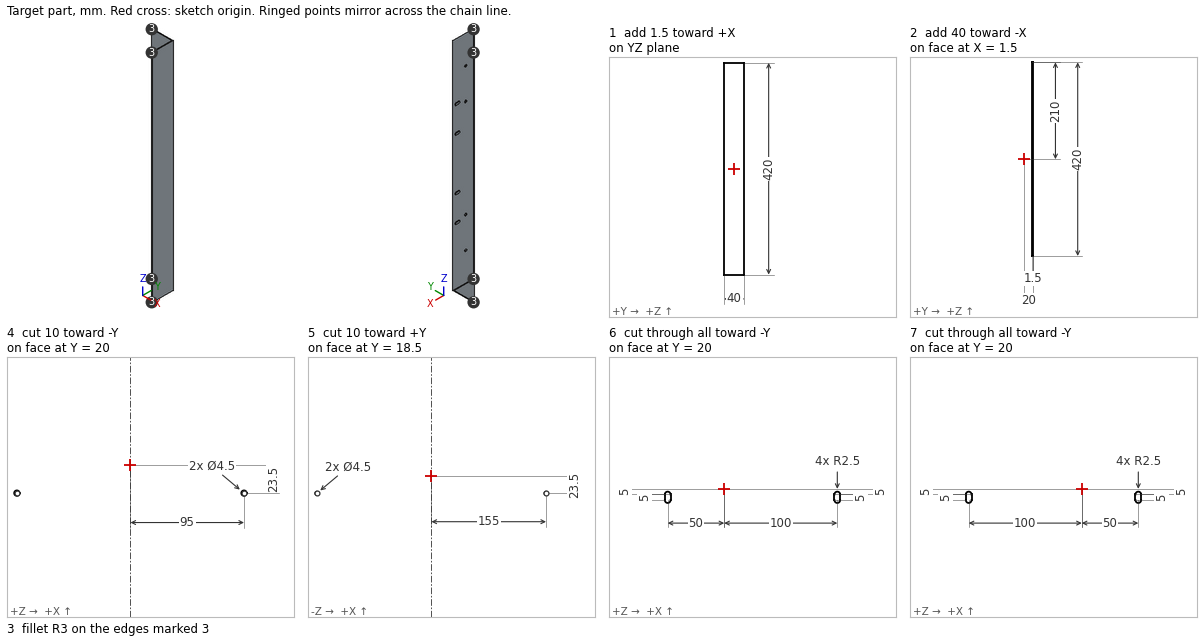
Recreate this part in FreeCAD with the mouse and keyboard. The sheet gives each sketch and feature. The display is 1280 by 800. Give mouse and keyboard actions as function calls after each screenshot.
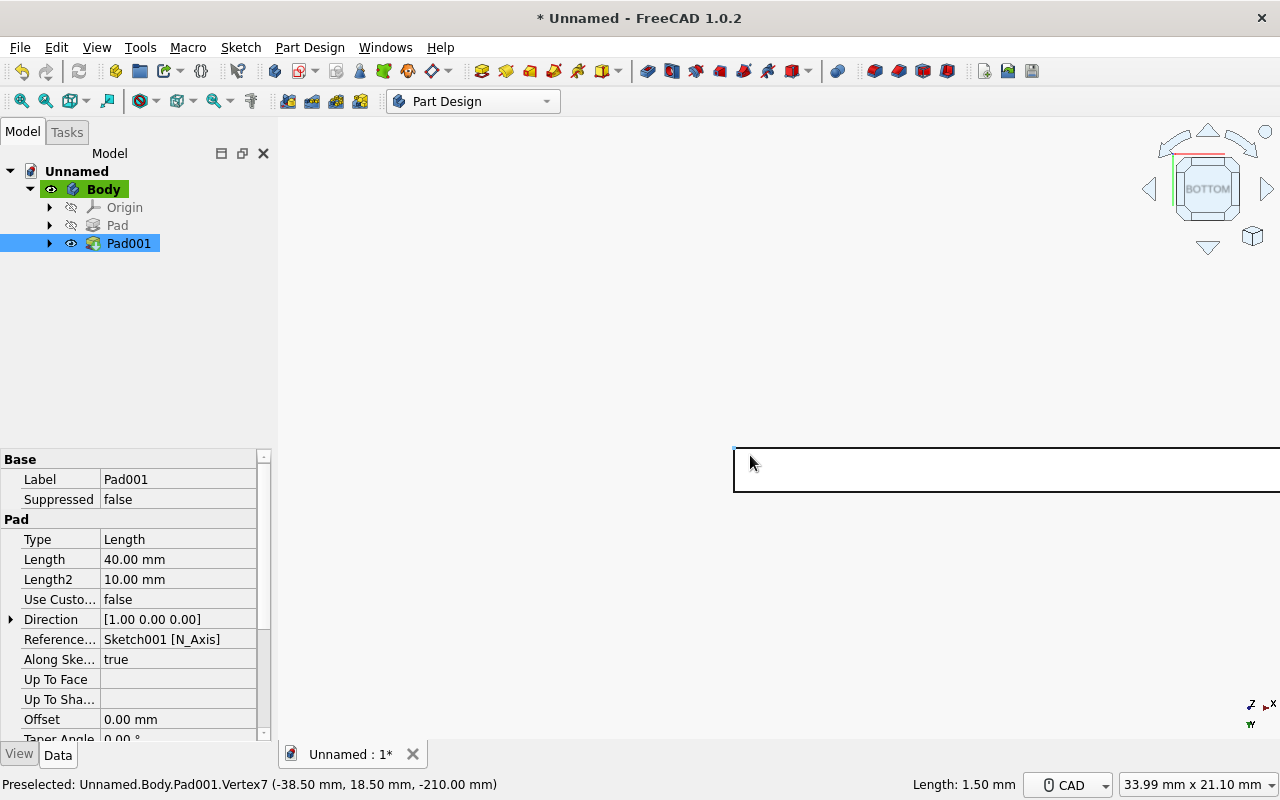
click(734, 469, ctrl)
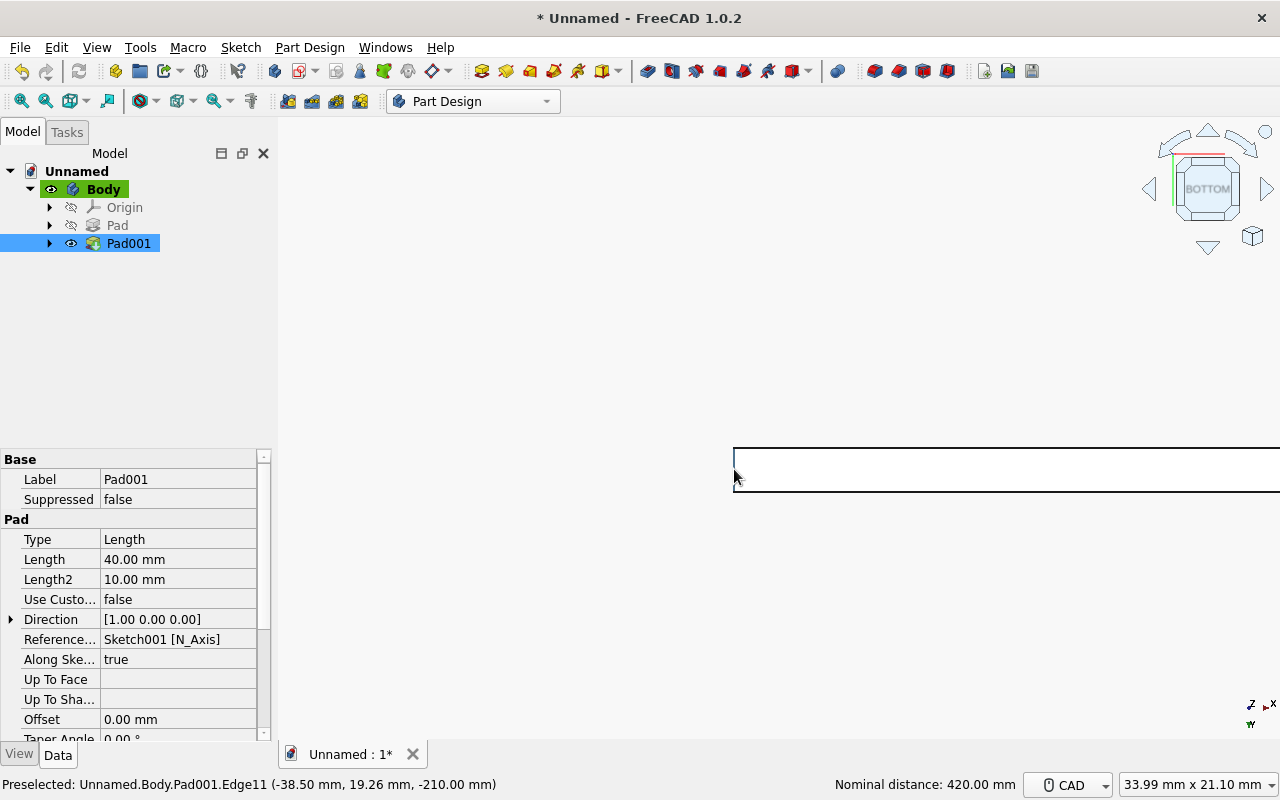
click(22, 102)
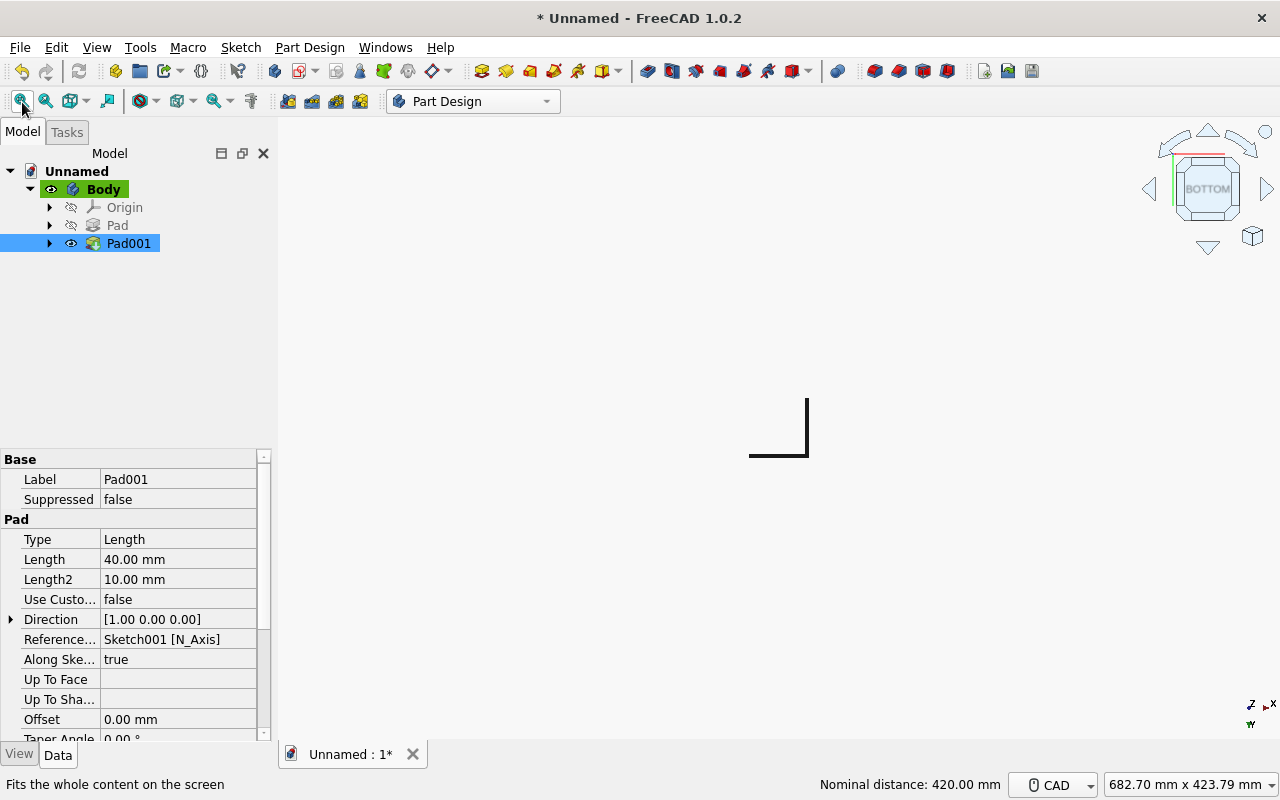
key(4)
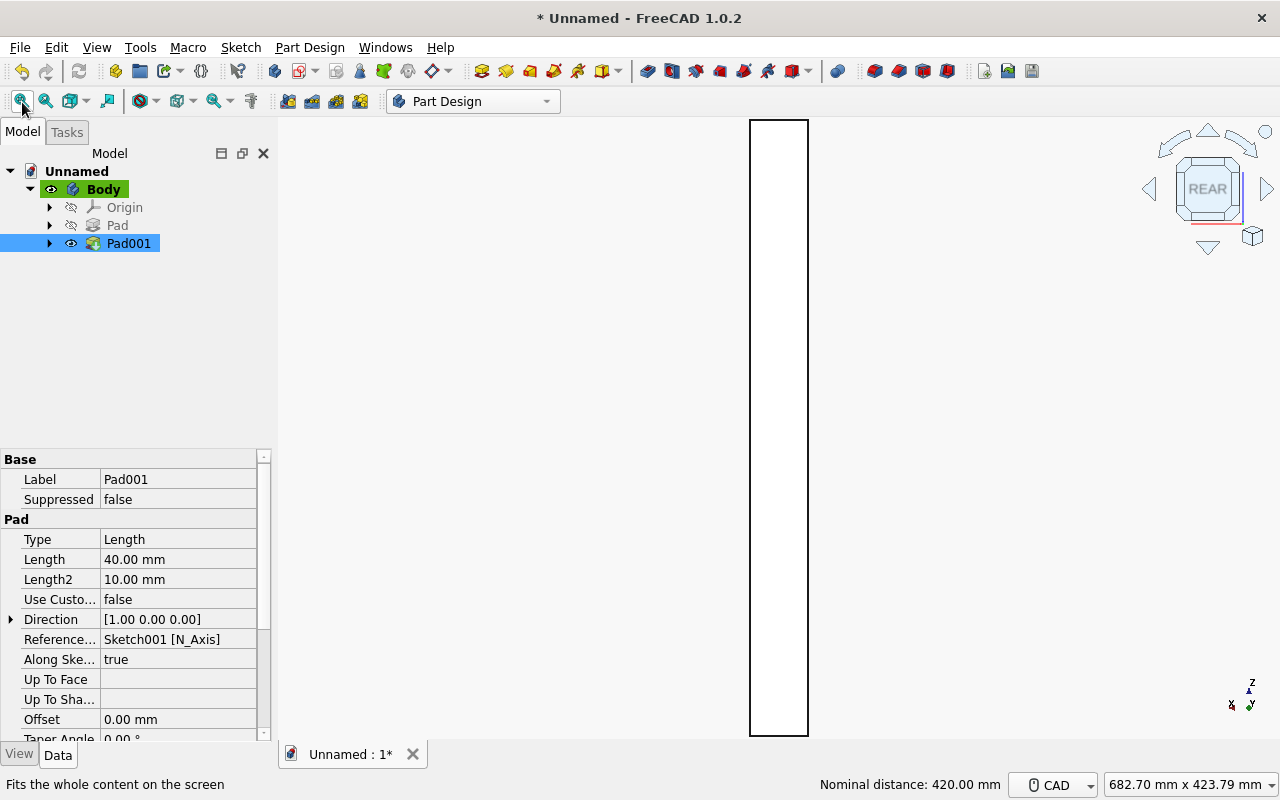
key(6)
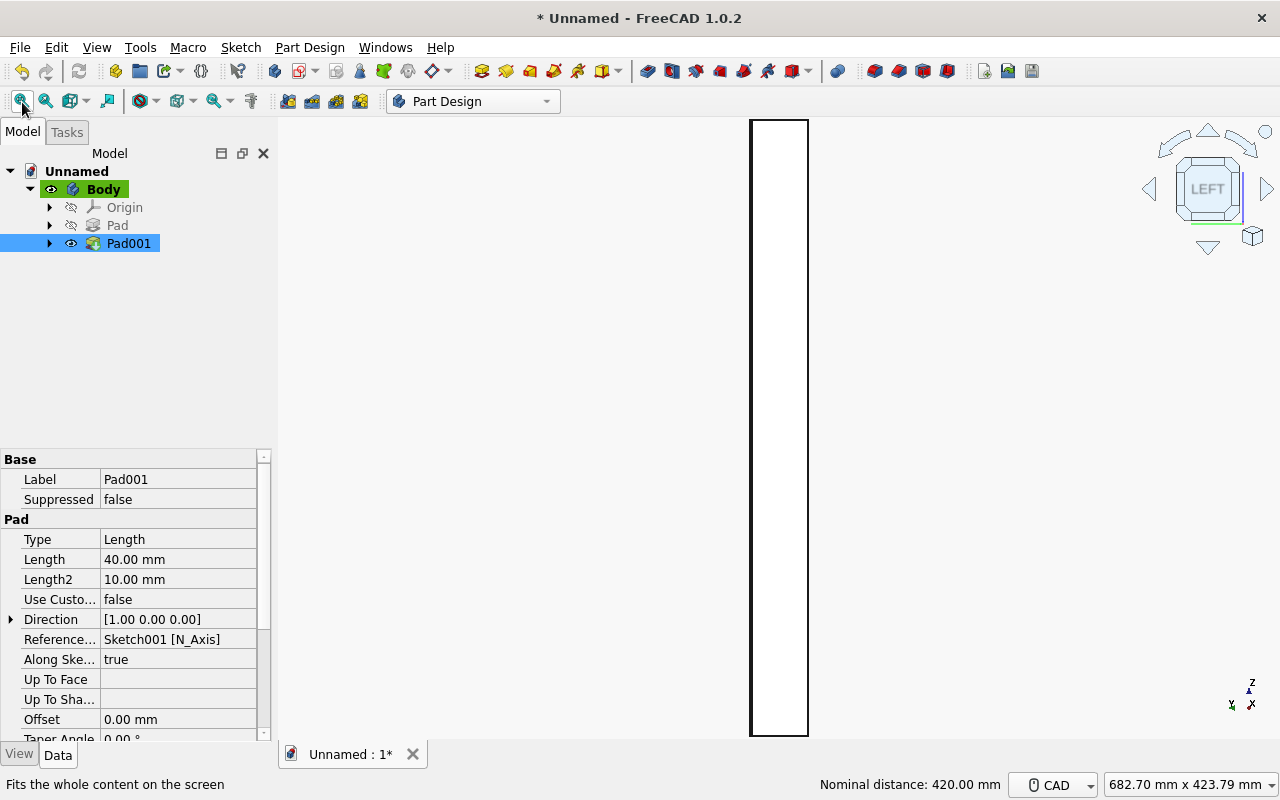
key(v)
key(3)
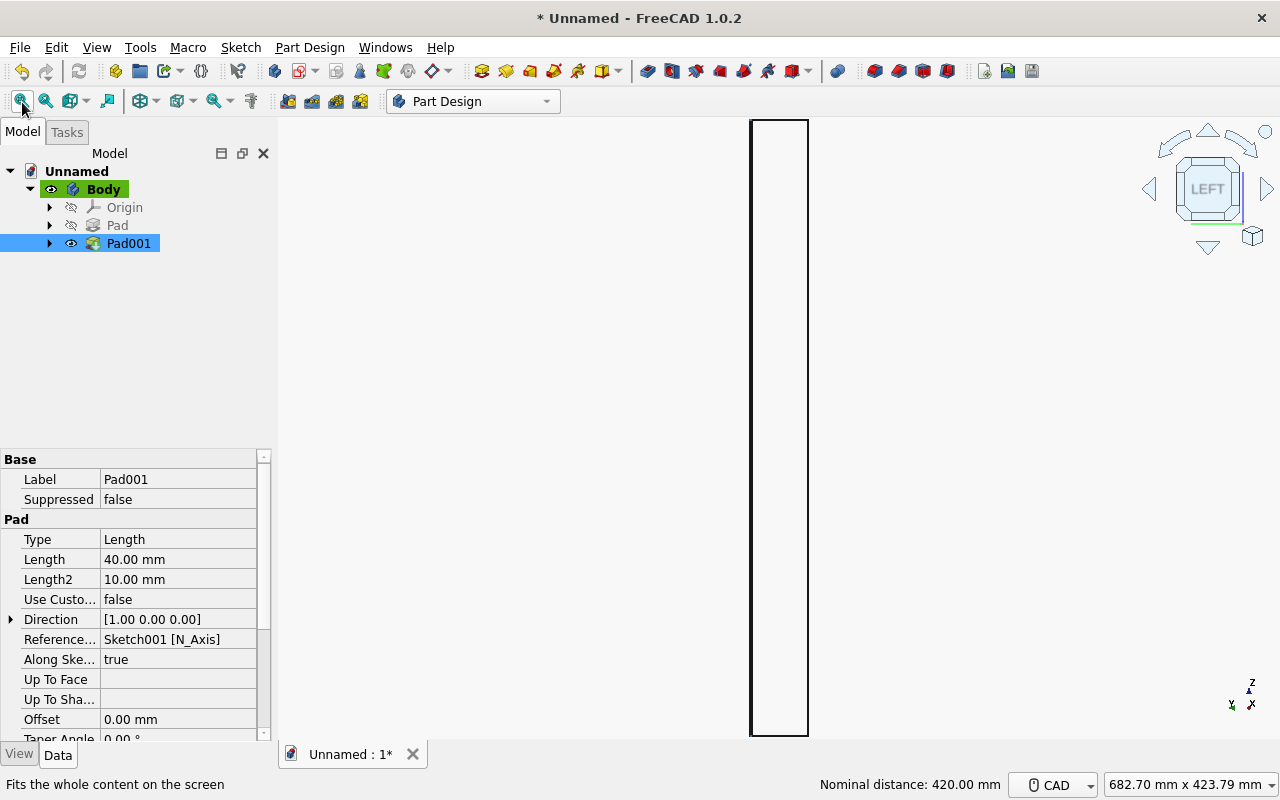
key(0)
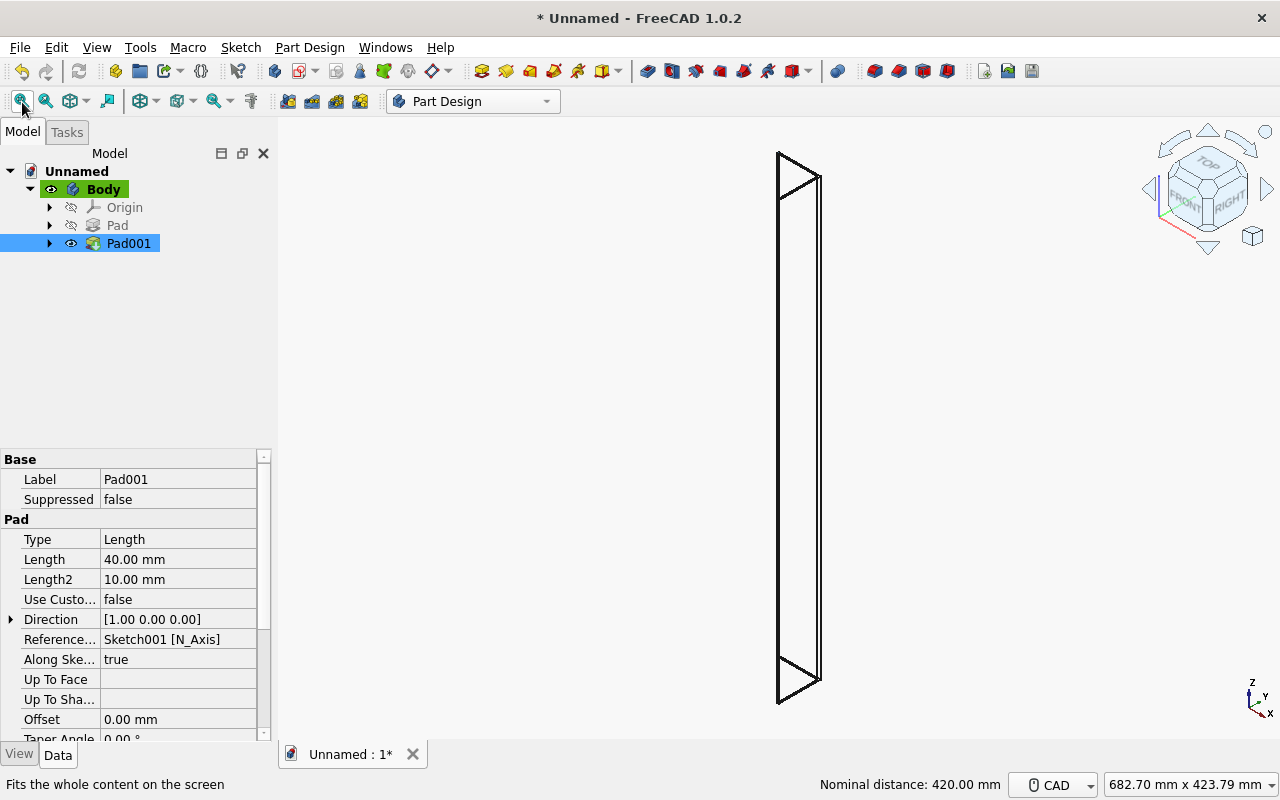
scroll(778, 702, up, 15)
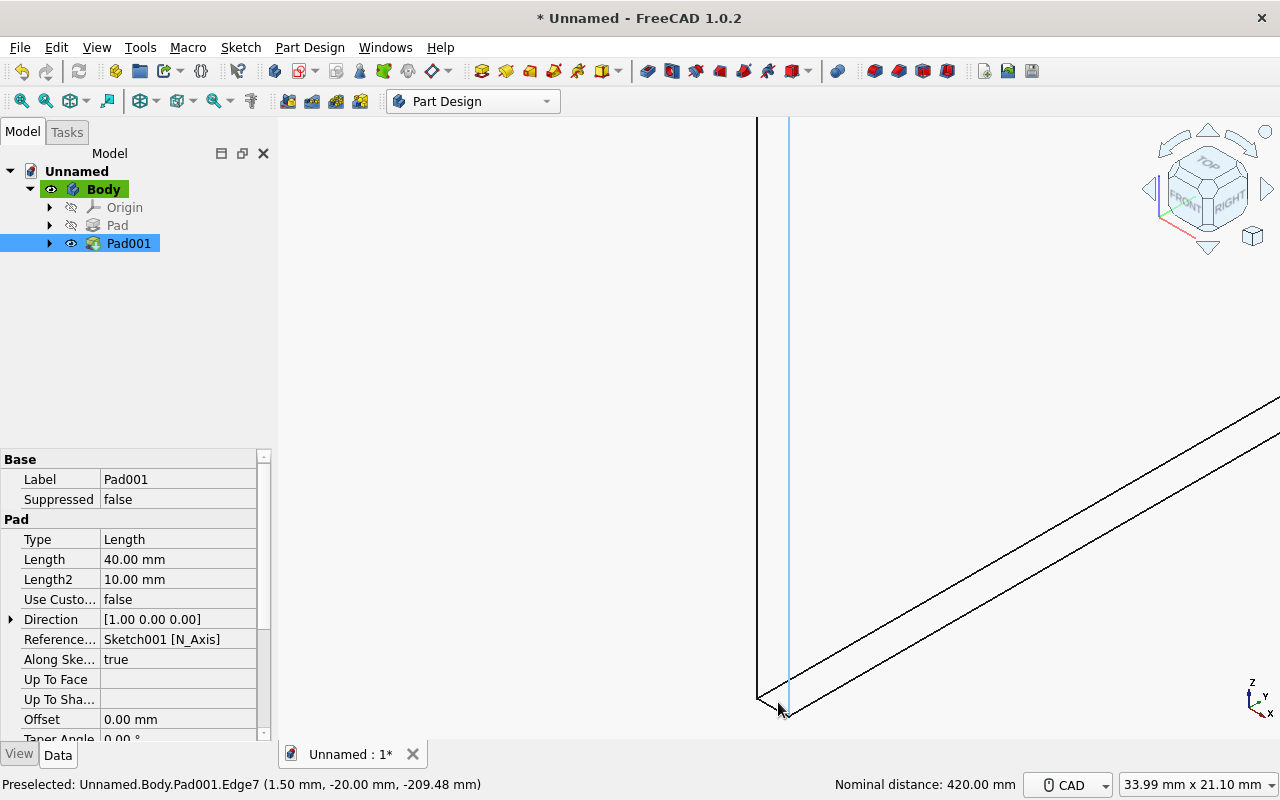
click(773, 707, ctrl)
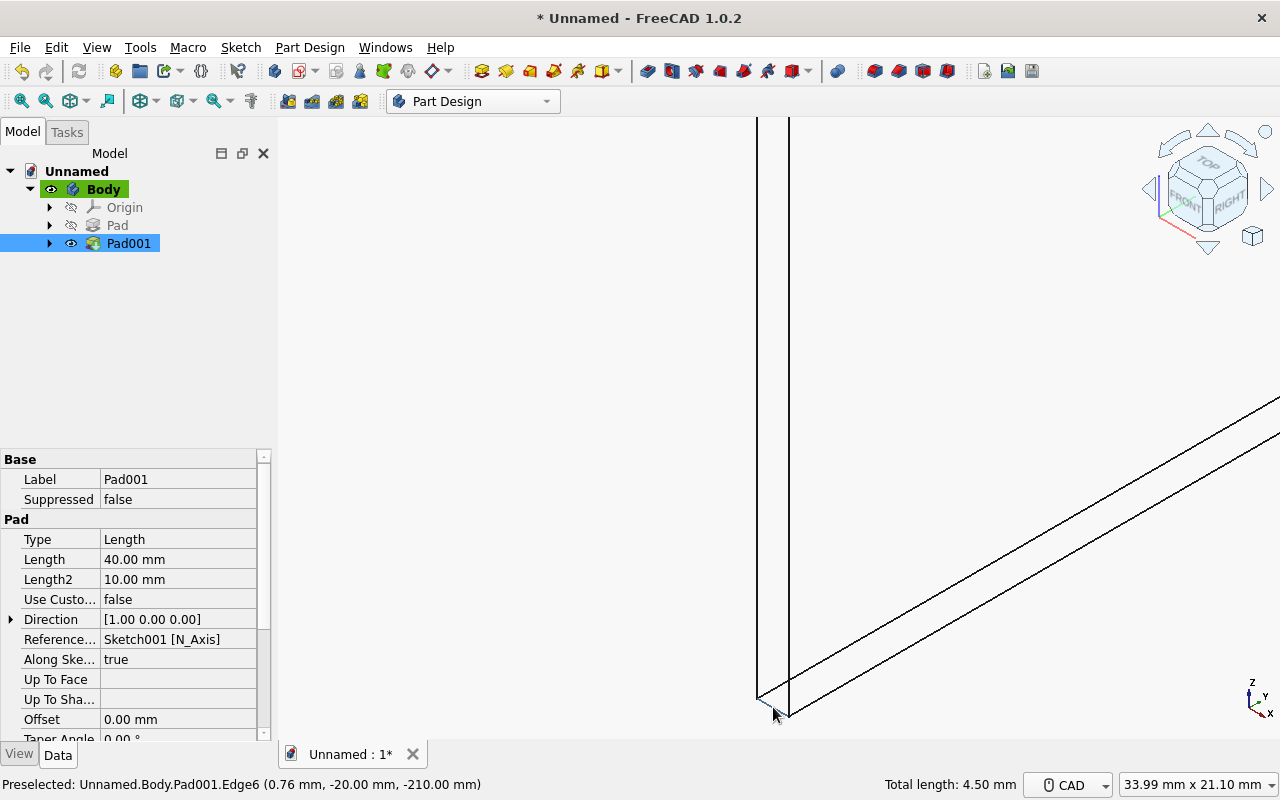
click(22, 102)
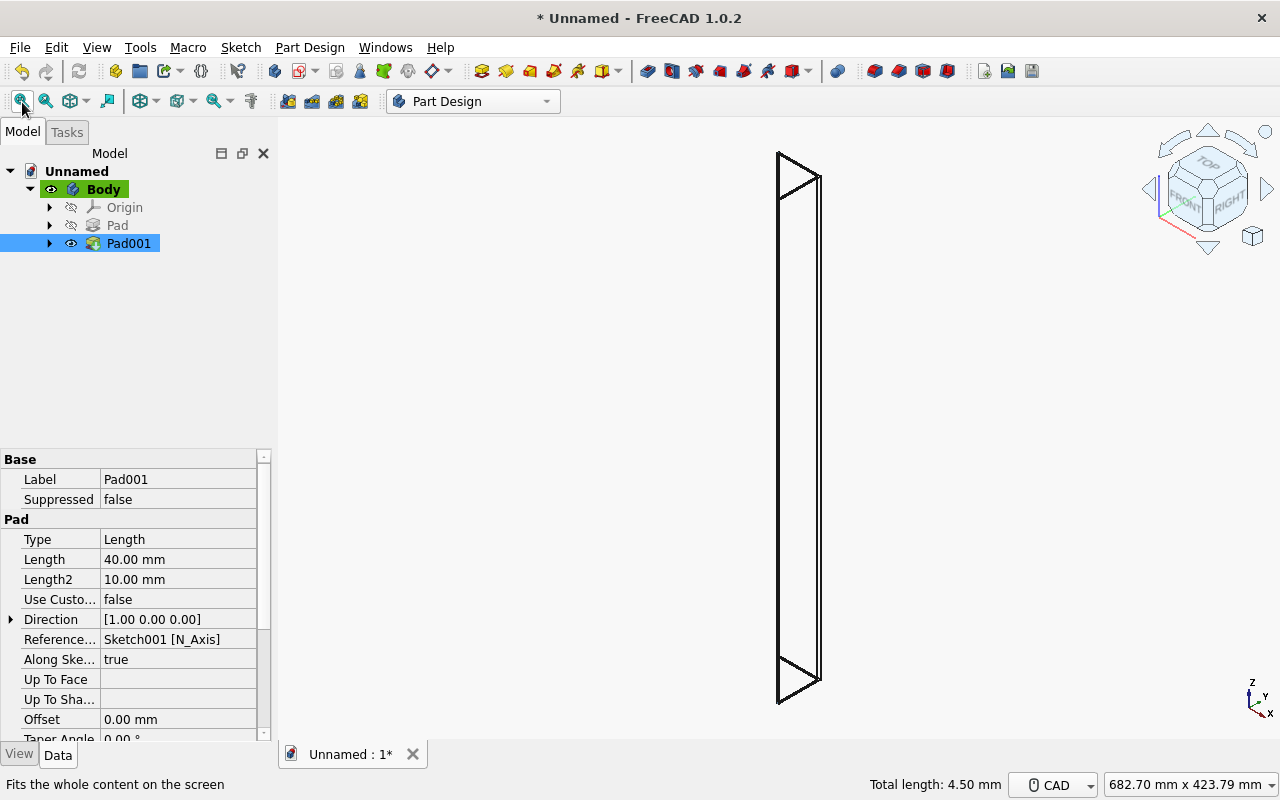
key(2)